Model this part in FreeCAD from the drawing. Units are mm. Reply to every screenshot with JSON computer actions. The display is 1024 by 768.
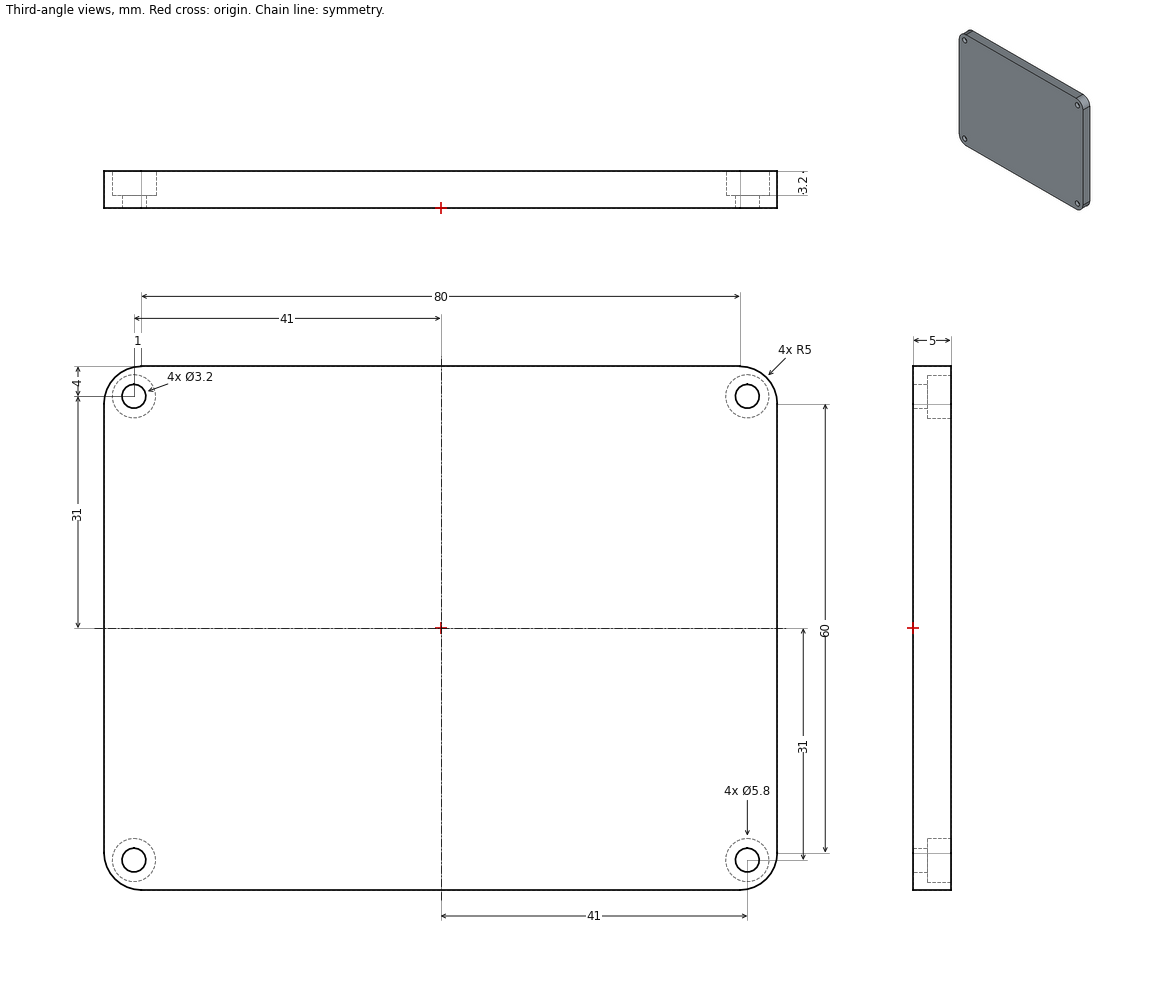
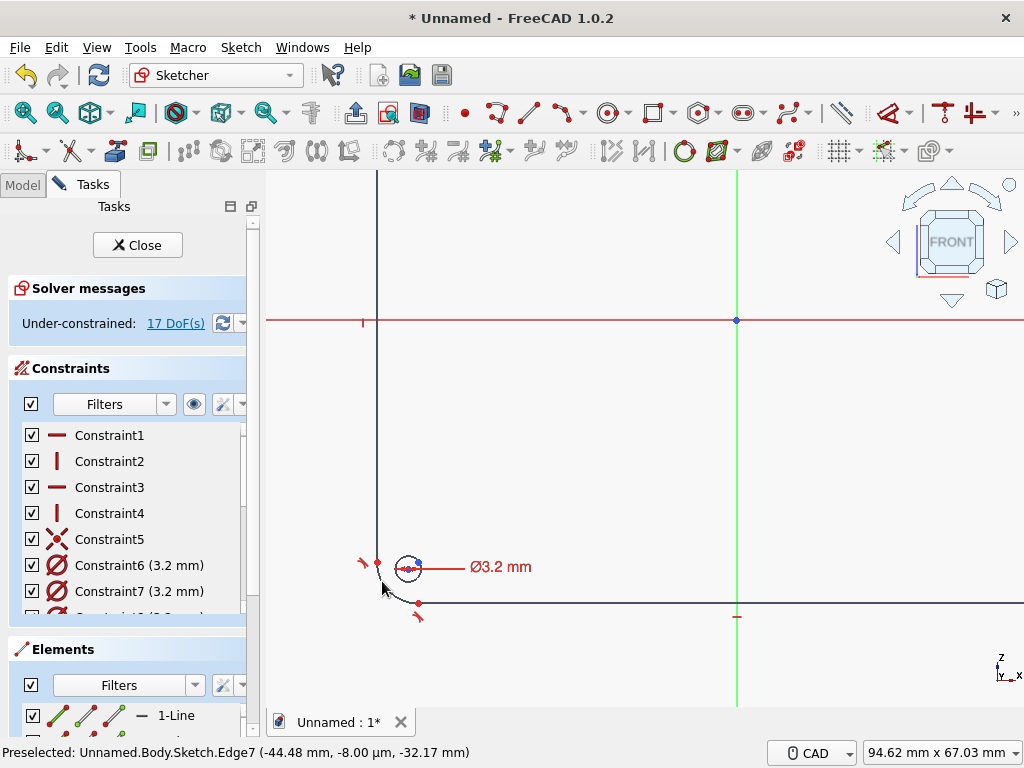
{"action": "left_click", "coordinate": [377, 418]}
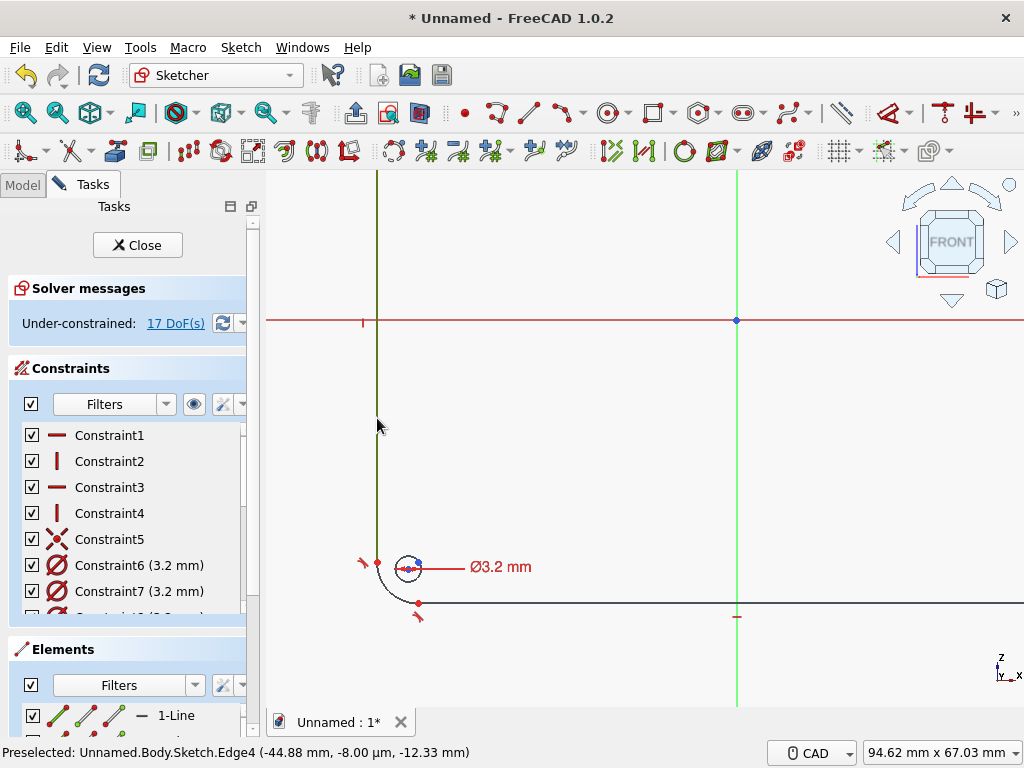
{"action": "scroll", "coordinate": [382, 582], "scroll_direction": "down", "scroll_amount": 3}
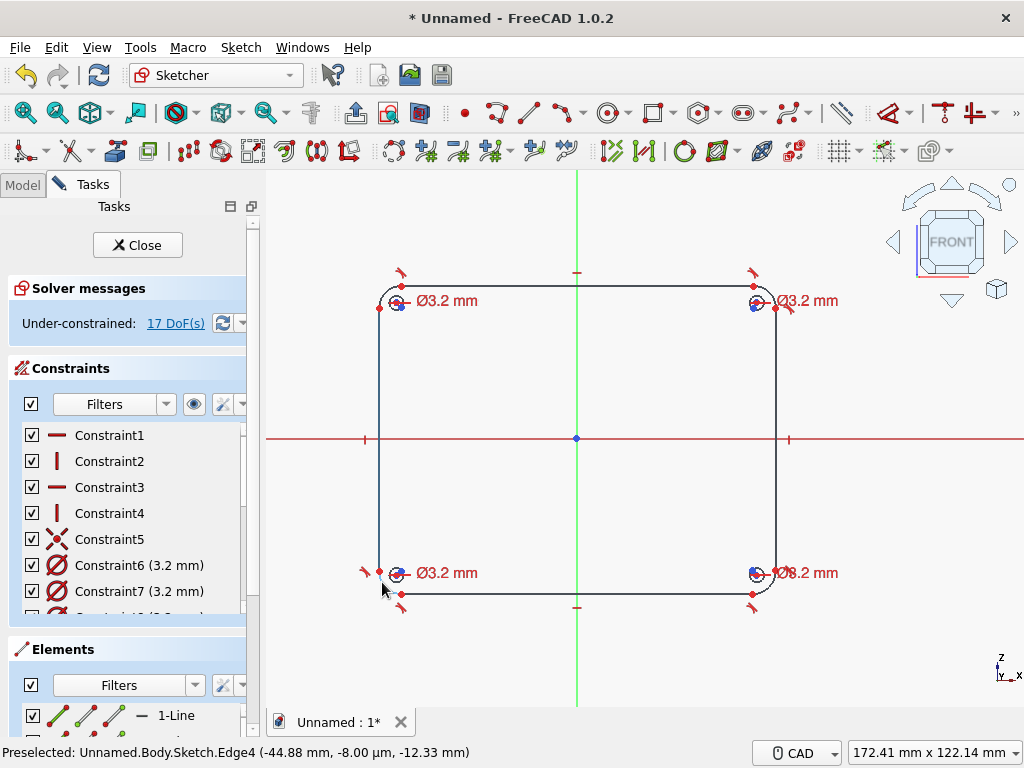
{"action": "scroll", "coordinate": [391, 288], "scroll_direction": "up", "scroll_amount": 3}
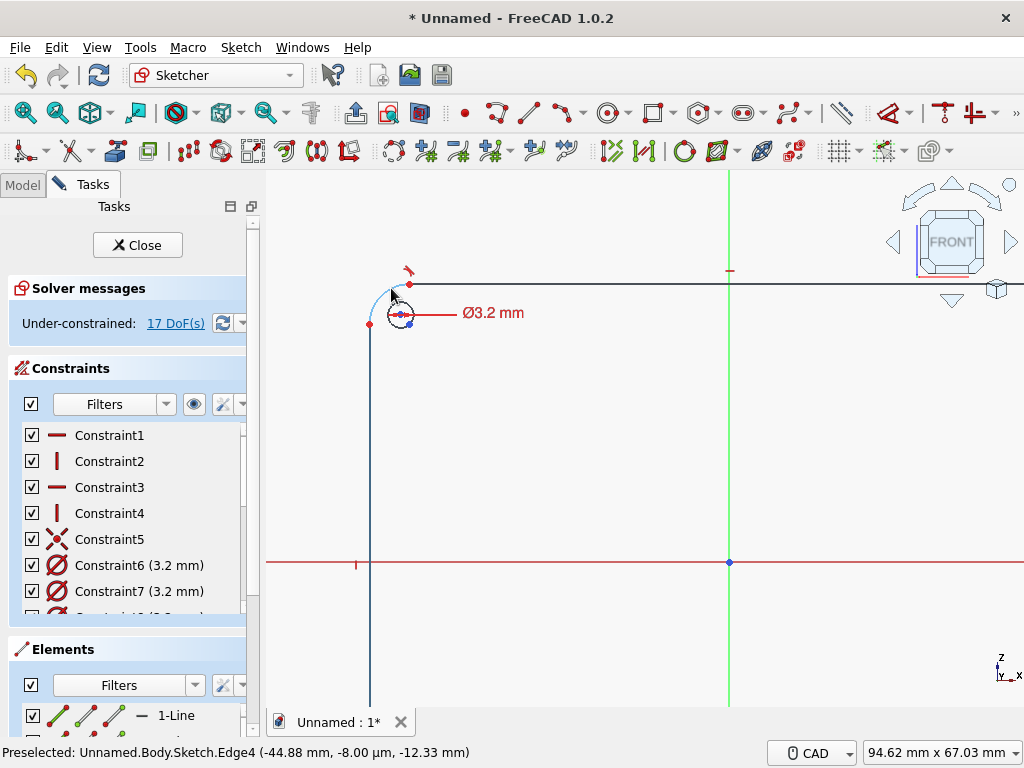
{"action": "left_click", "coordinate": [391, 289]}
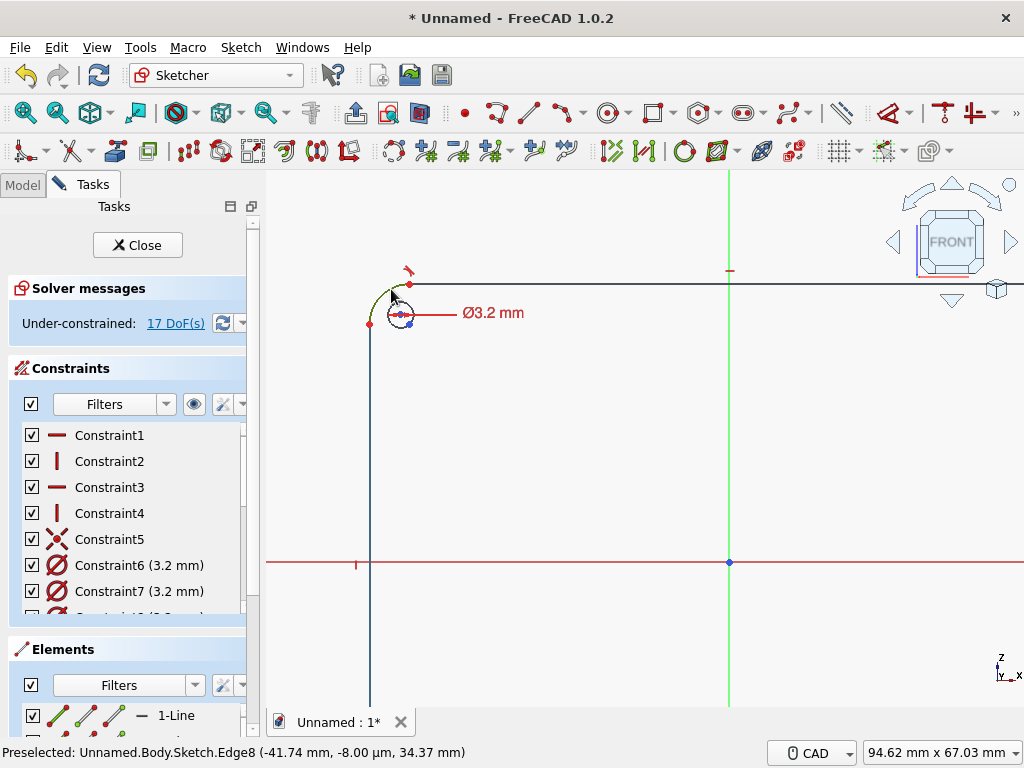
{"action": "key", "text": "t"}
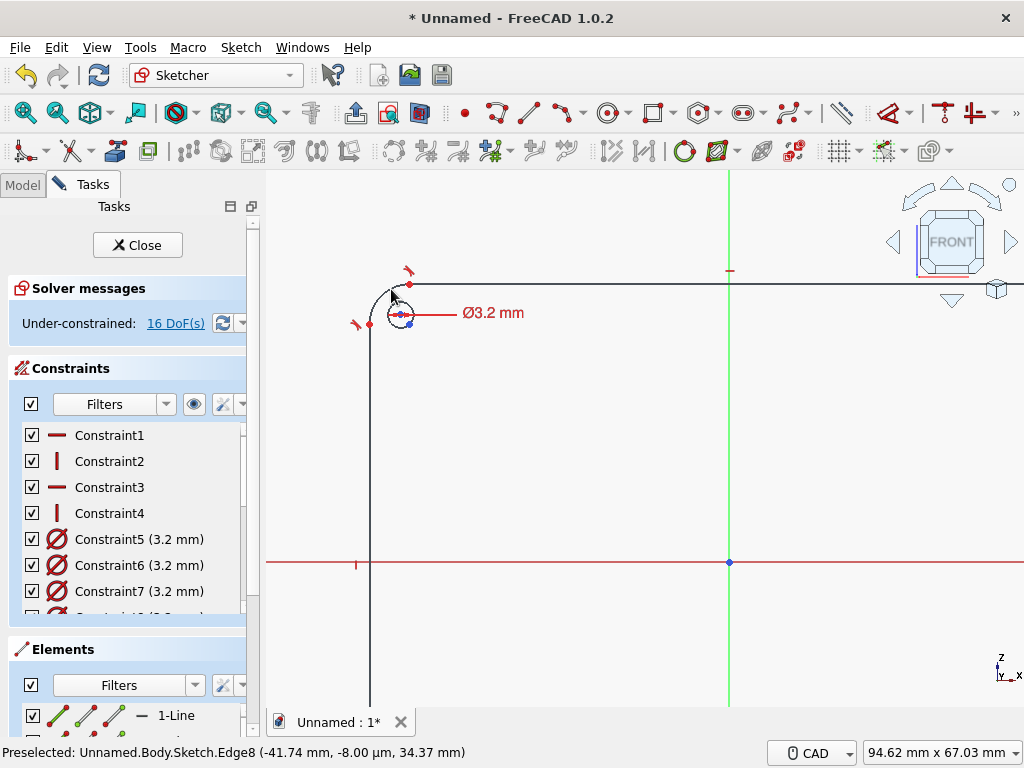
{"action": "scroll", "coordinate": [391, 288], "scroll_direction": "down", "scroll_amount": 3}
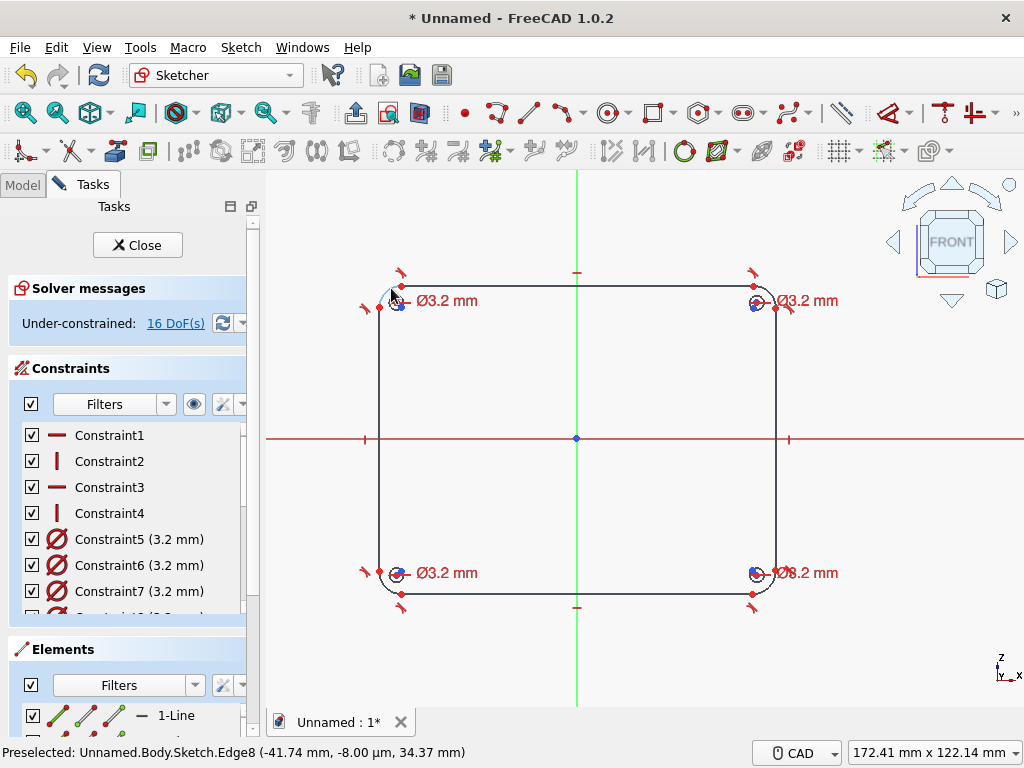
{"action": "scroll", "coordinate": [773, 298], "scroll_direction": "up", "scroll_amount": 2}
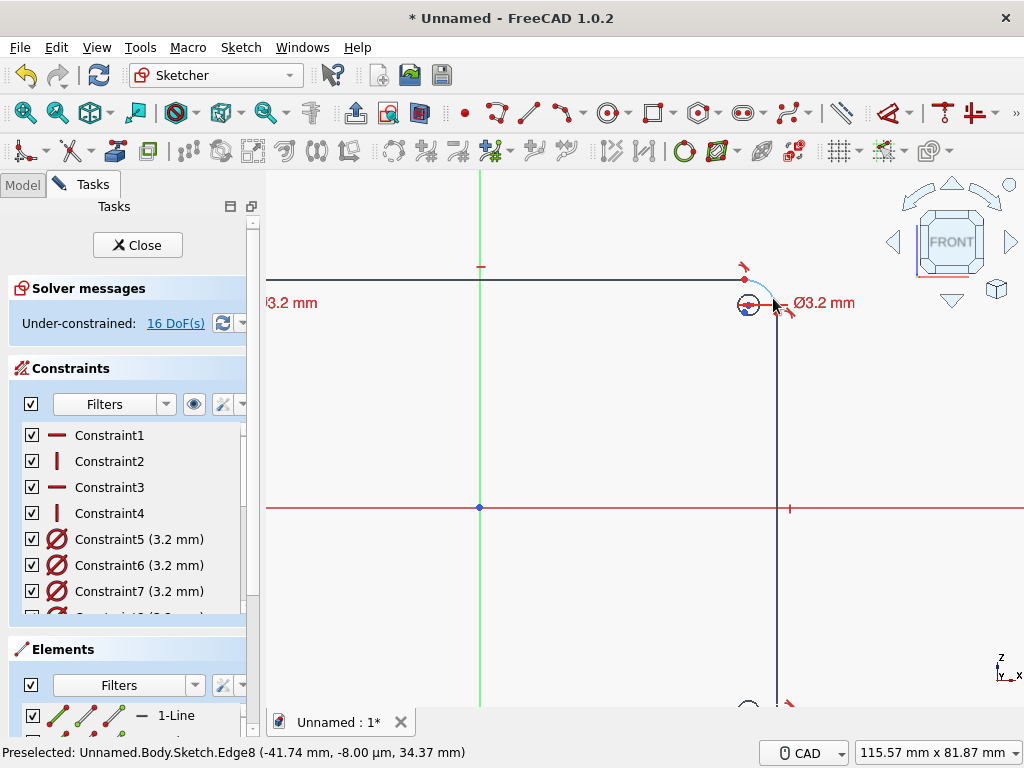
{"action": "left_click", "coordinate": [773, 298]}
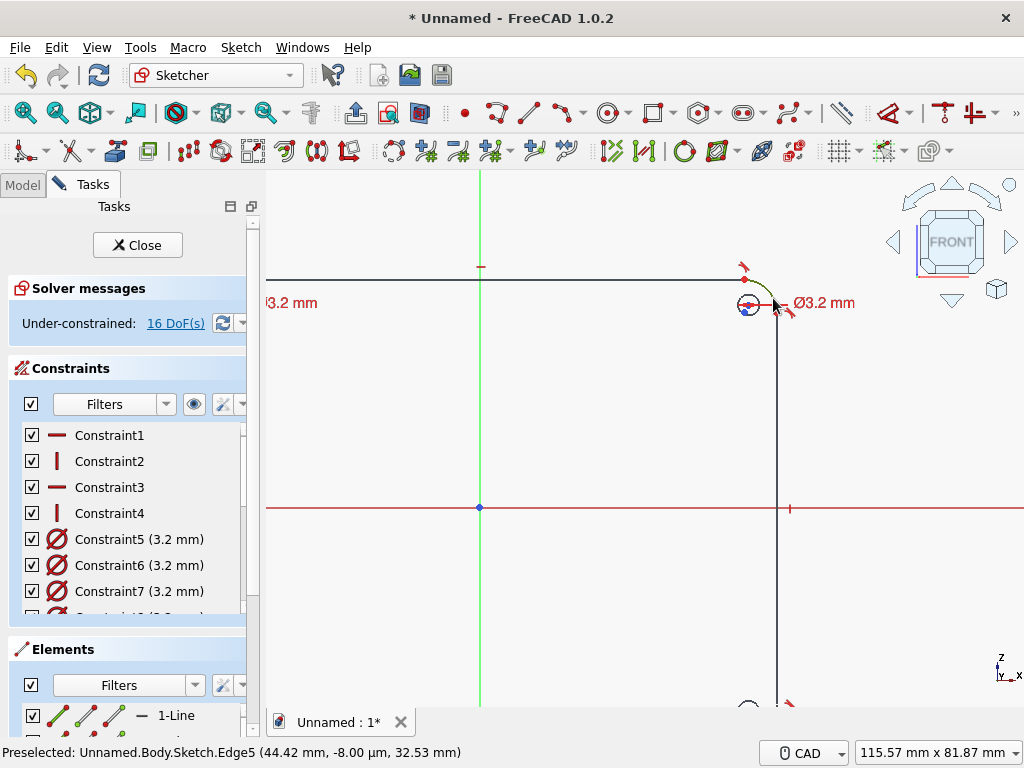
{"action": "scroll", "coordinate": [773, 298], "scroll_direction": "down", "scroll_amount": 2}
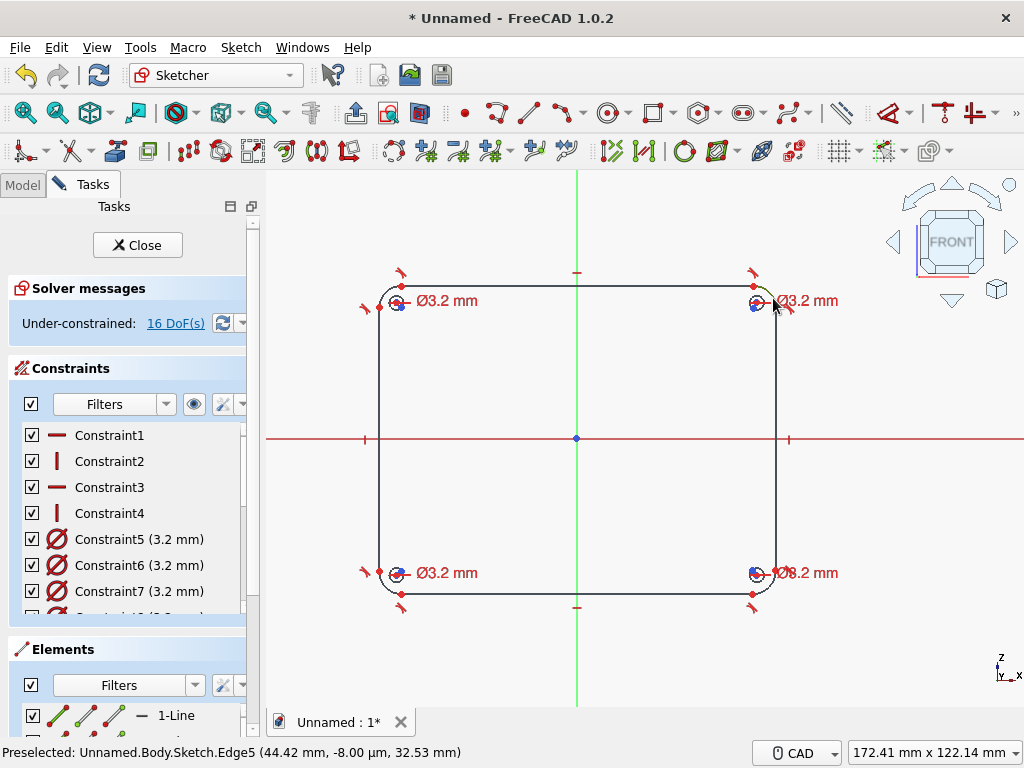
{"action": "scroll", "coordinate": [763, 592], "scroll_direction": "up", "scroll_amount": 2}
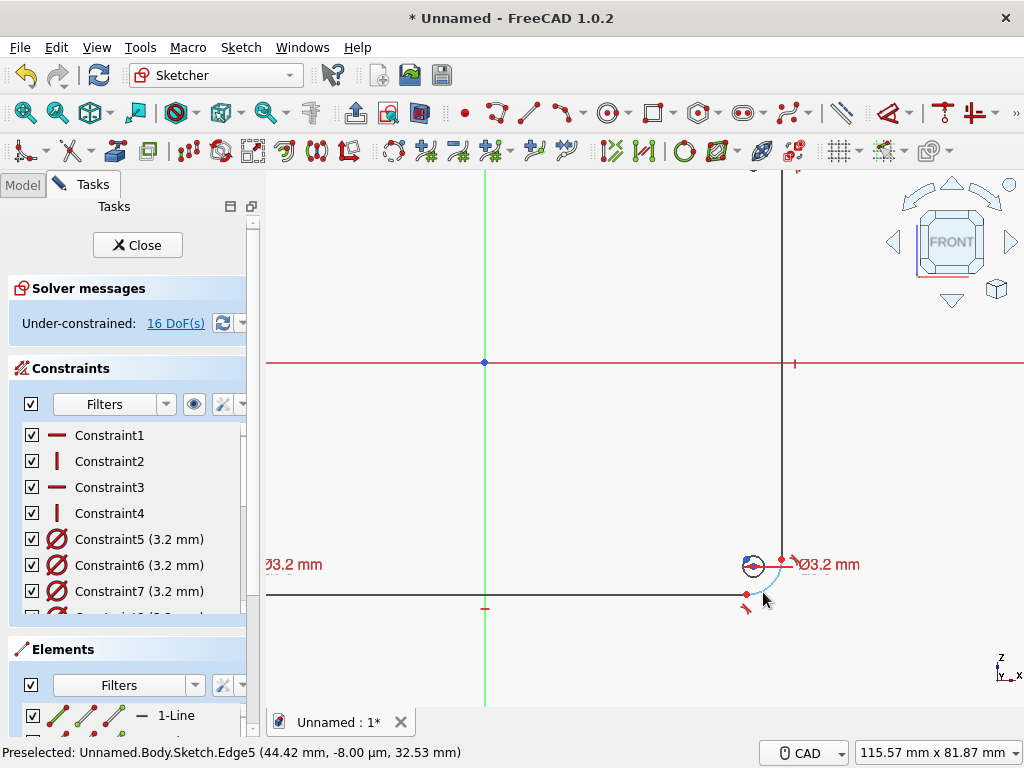
{"action": "left_click", "coordinate": [763, 591]}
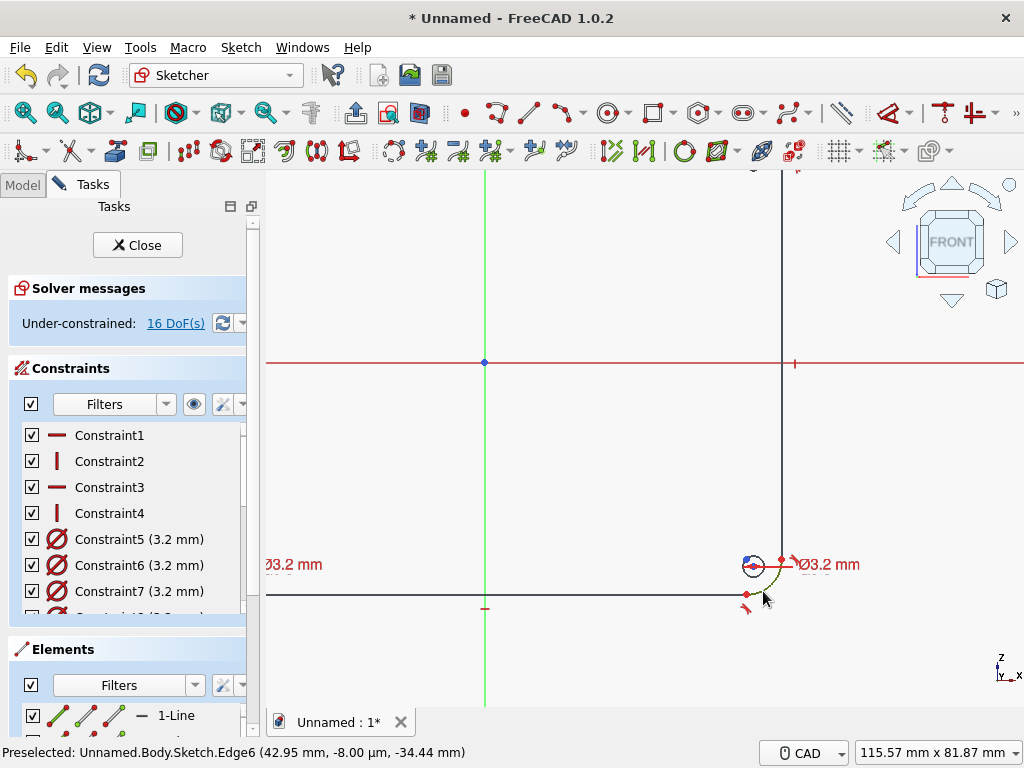
{"action": "scroll", "coordinate": [763, 592], "scroll_direction": "down", "scroll_amount": 2}